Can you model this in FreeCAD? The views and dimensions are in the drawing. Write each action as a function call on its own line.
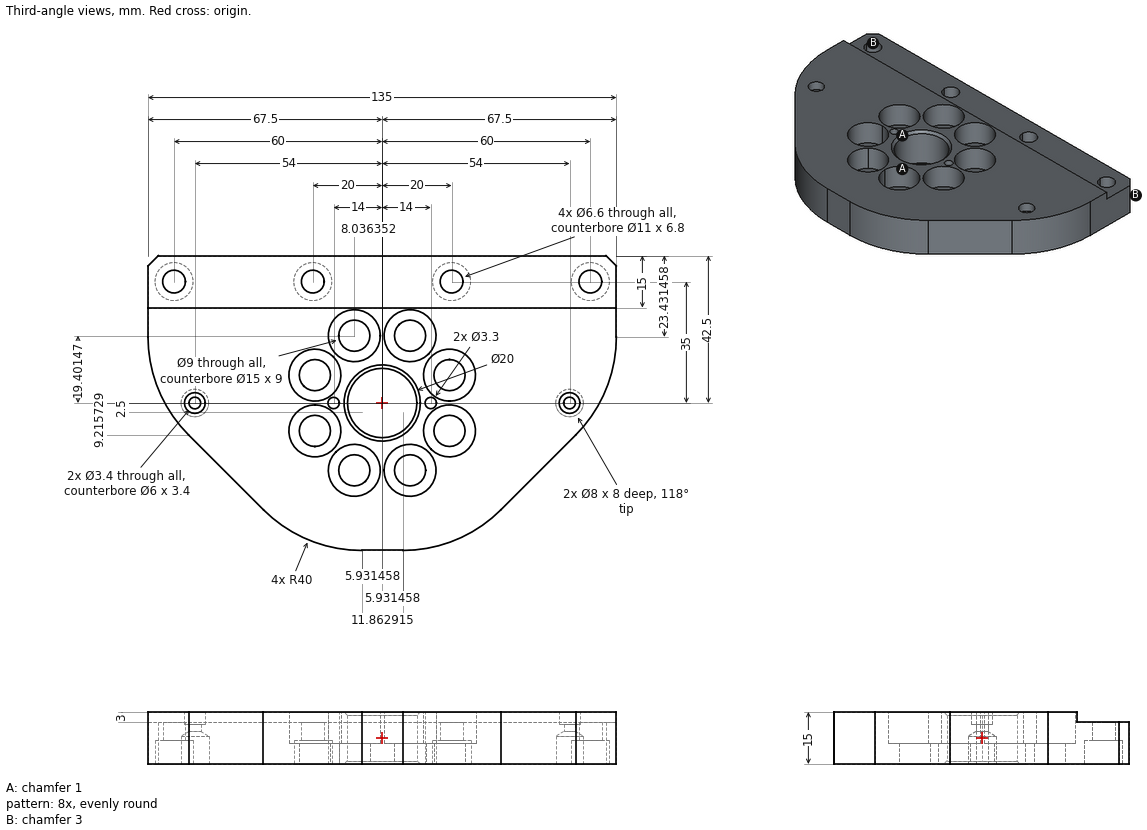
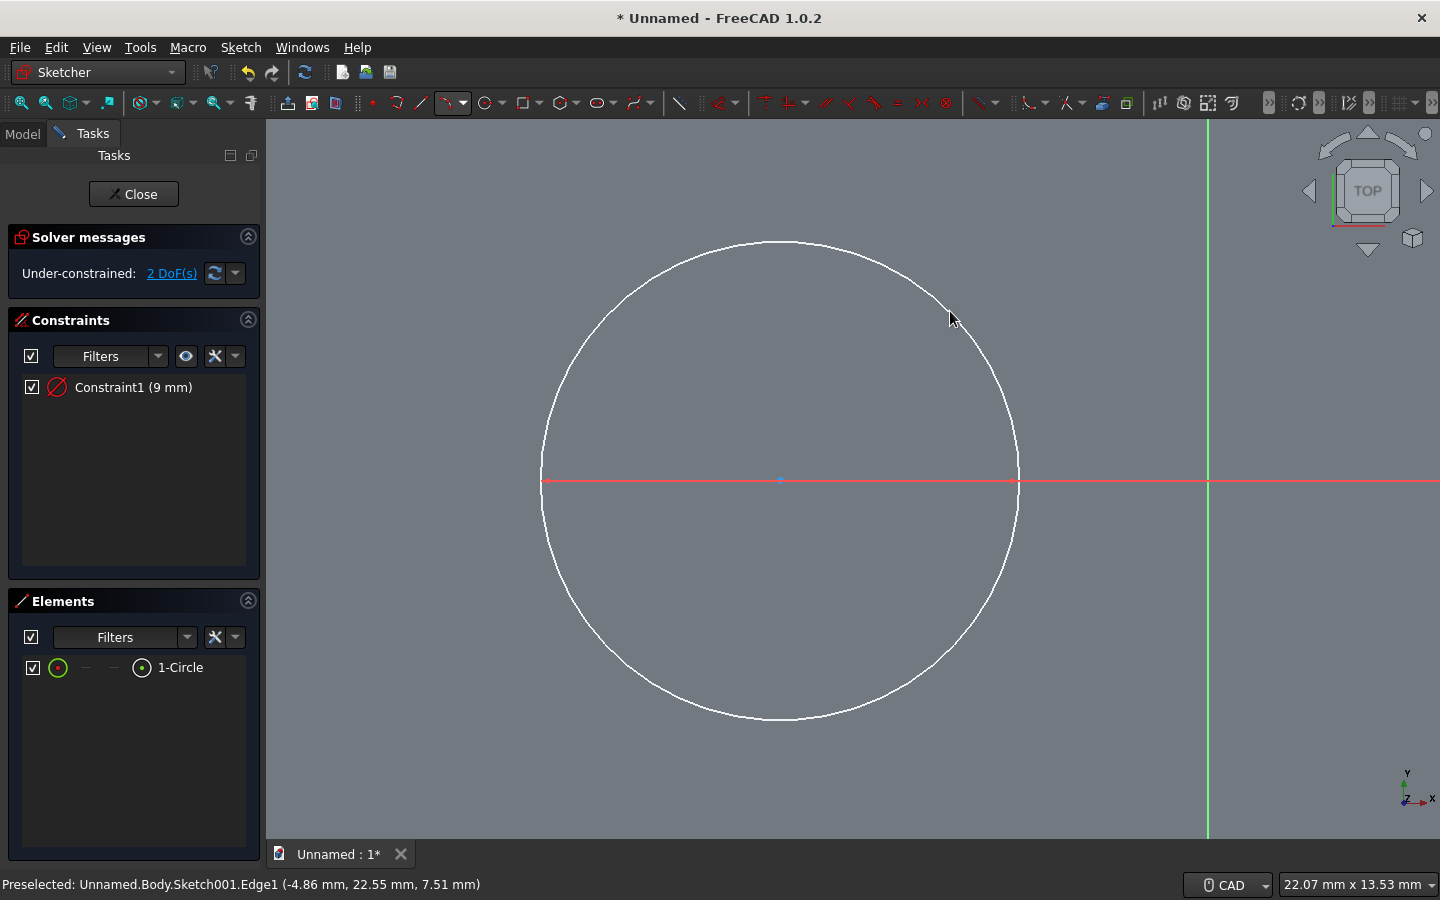
click(718, 104)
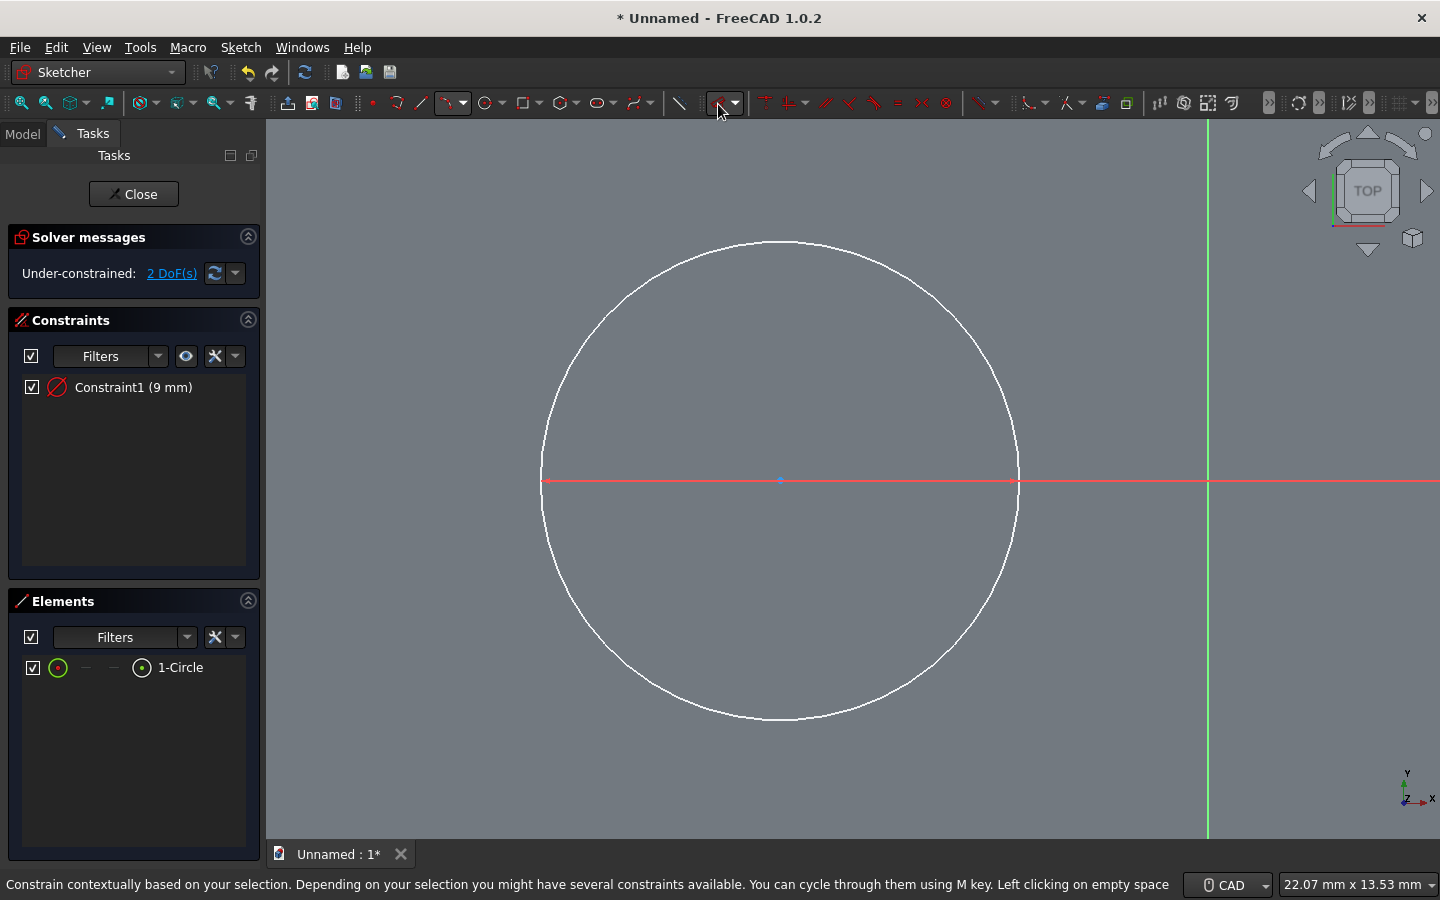
click(780, 481)
click(994, 447)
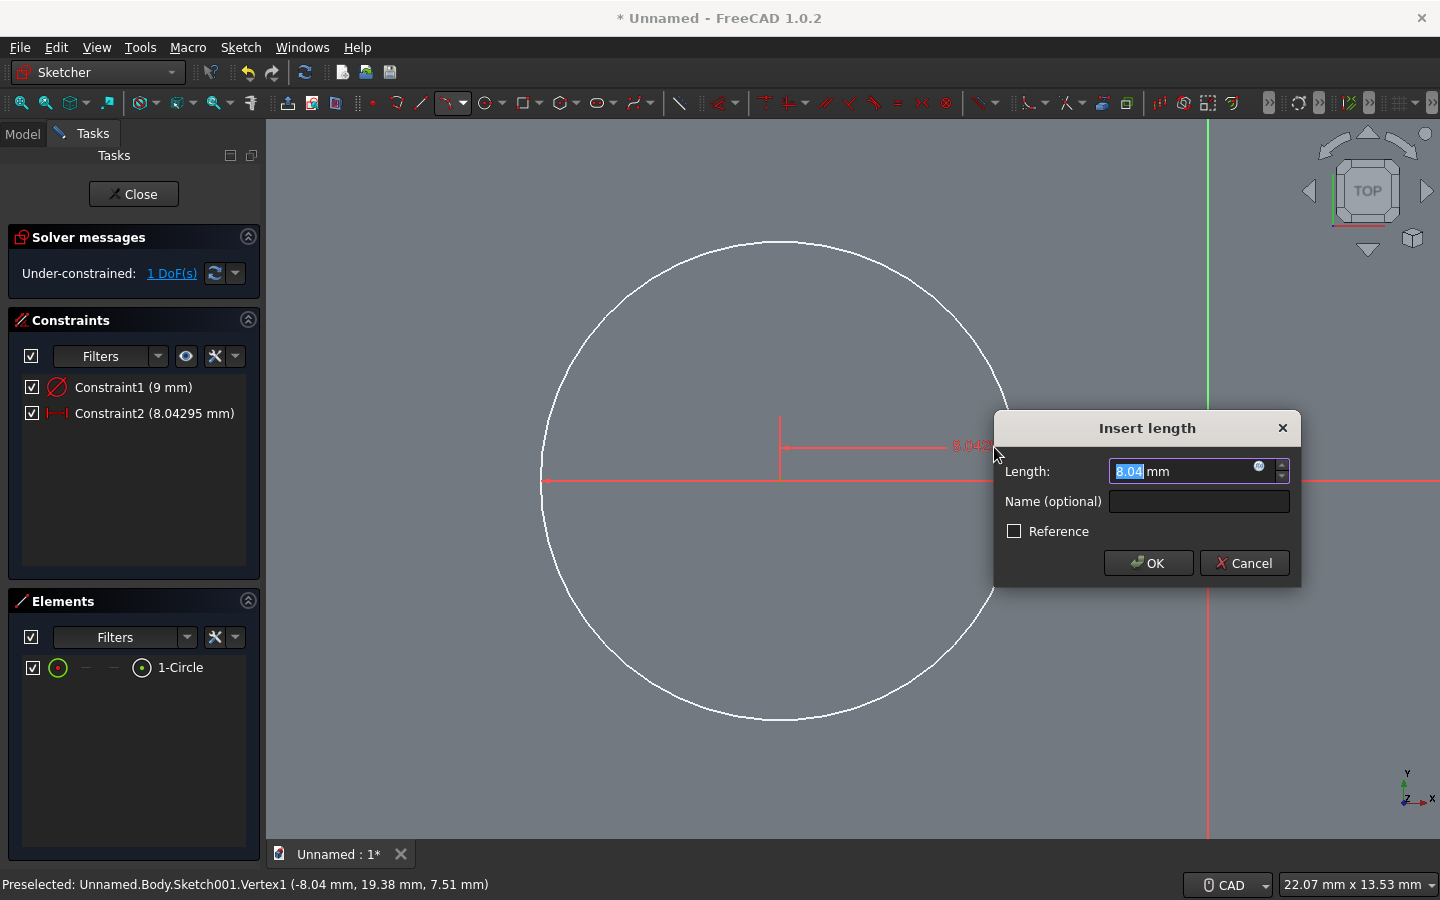
text(8.036352)
key(Return)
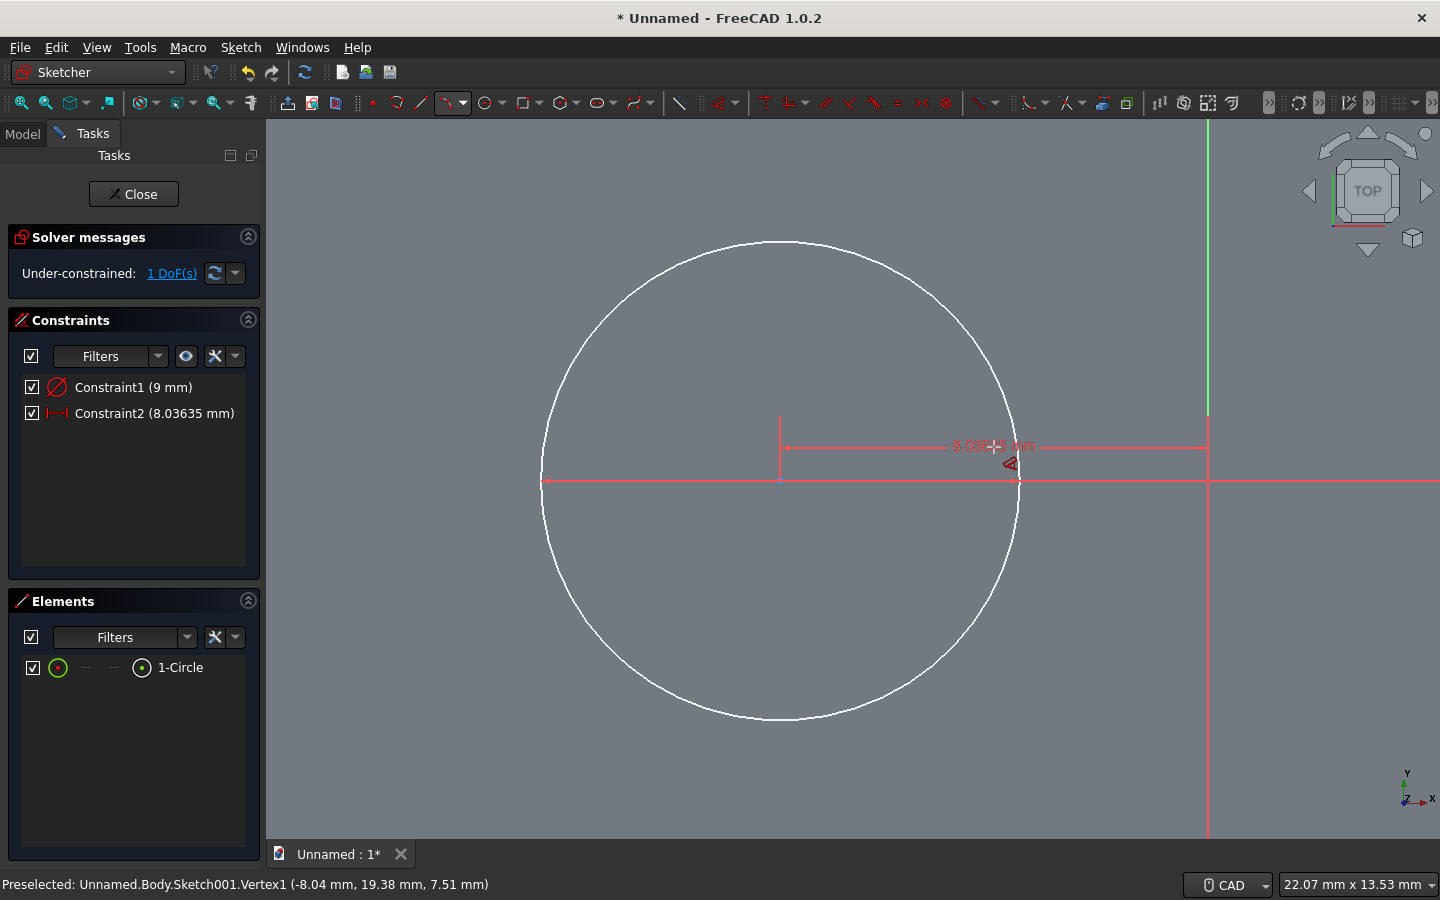
click(780, 481)
click(1242, 646)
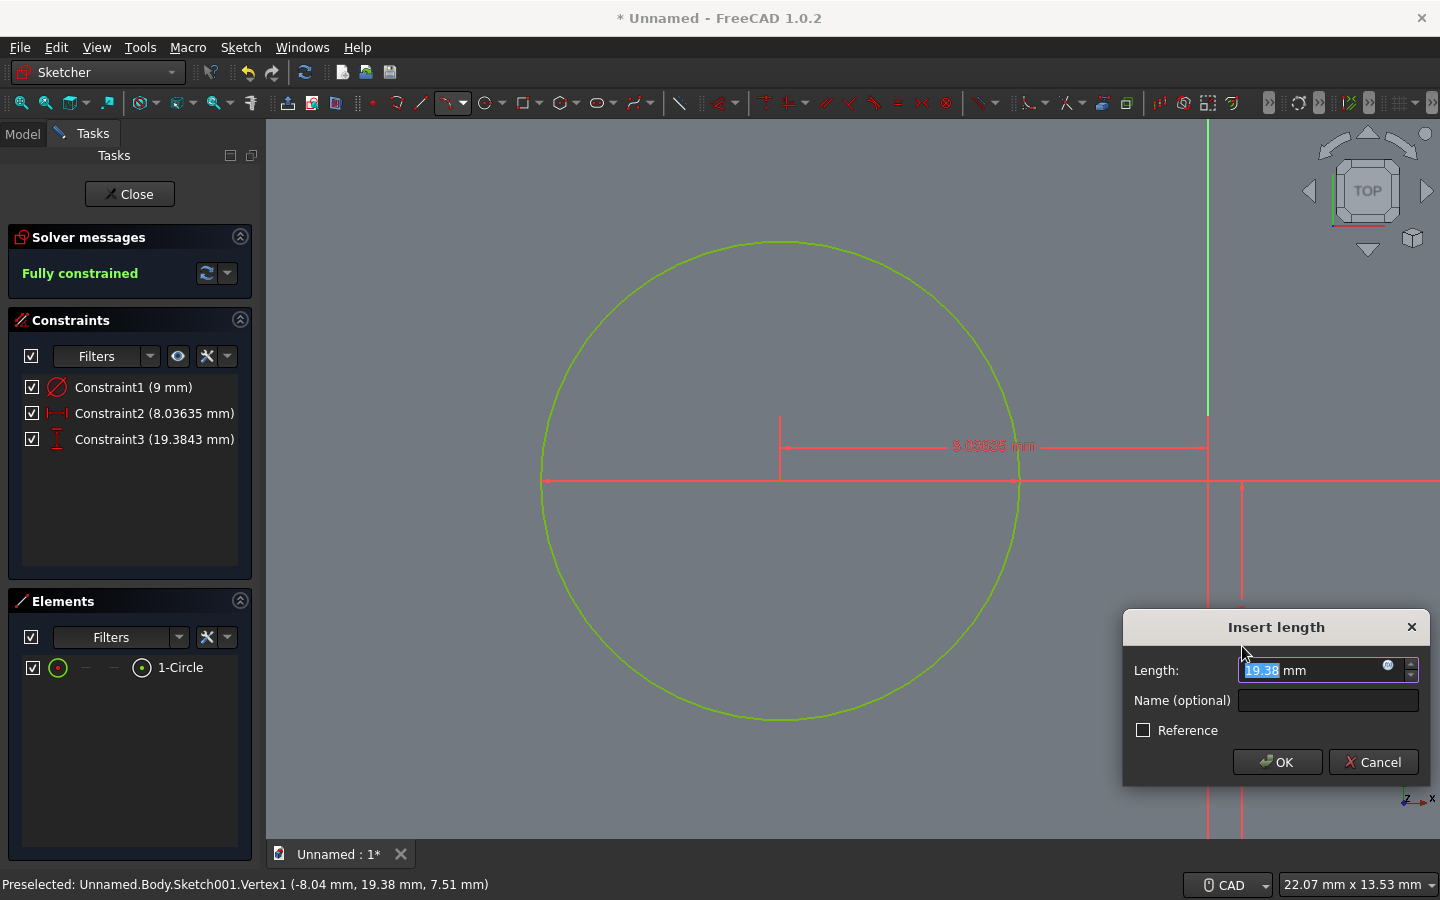
text(19.40147)
key(Return)
key(Escape)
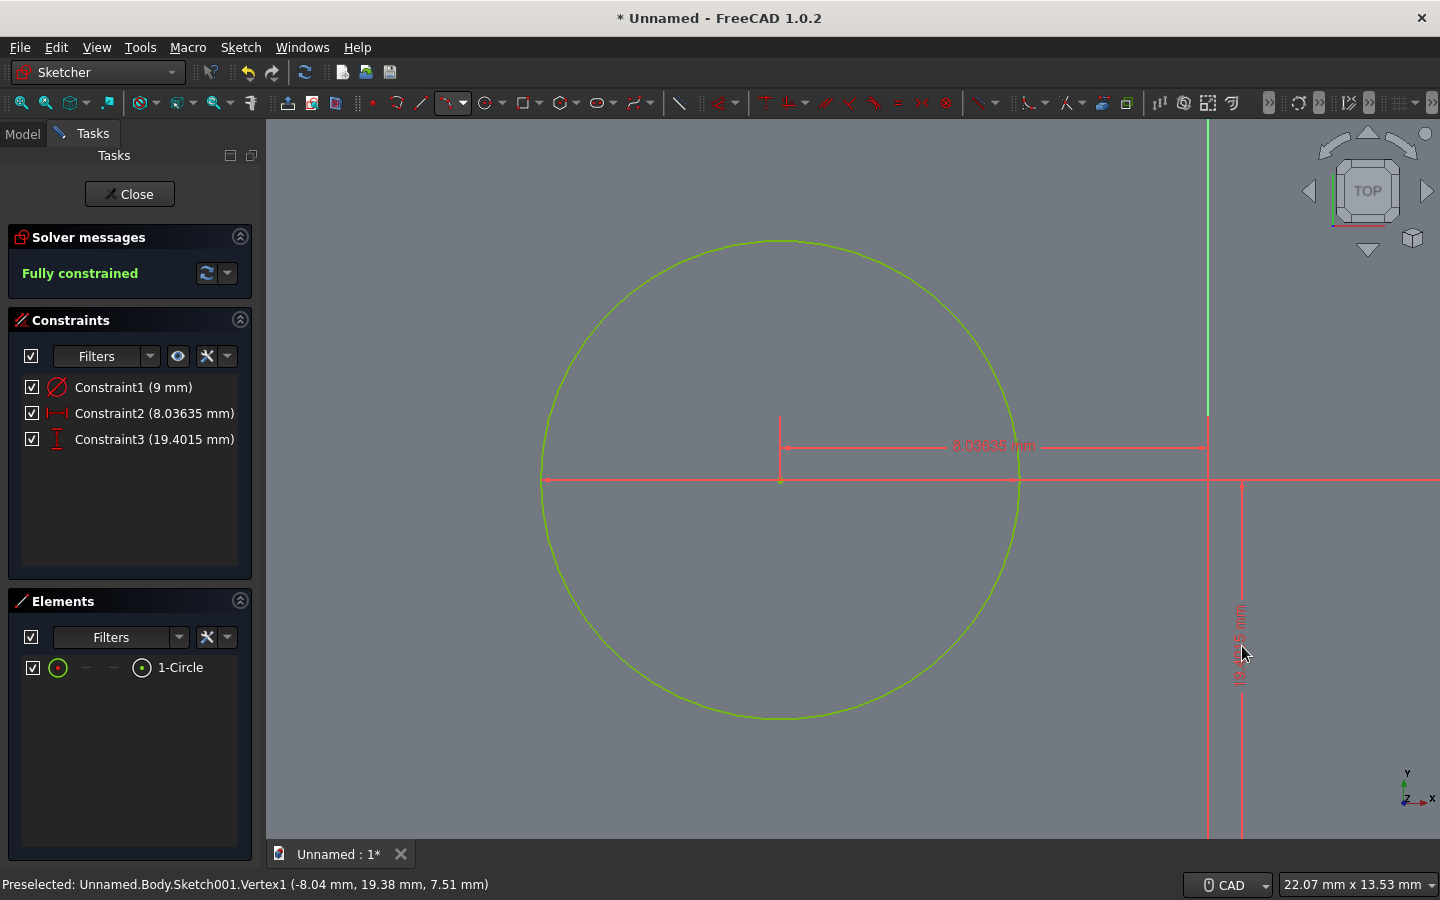
click(130, 194)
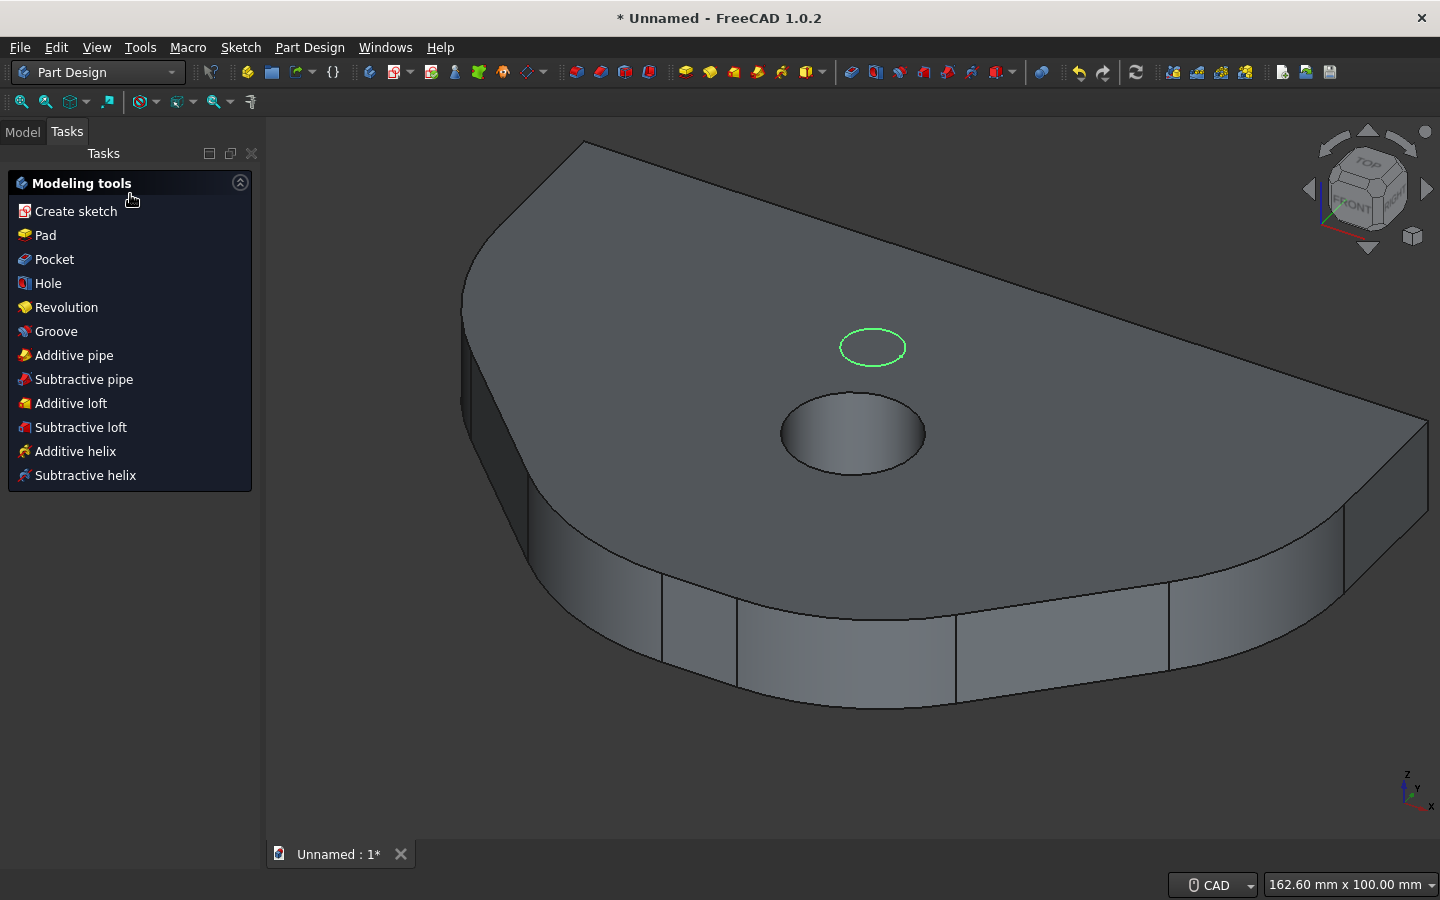
click(876, 72)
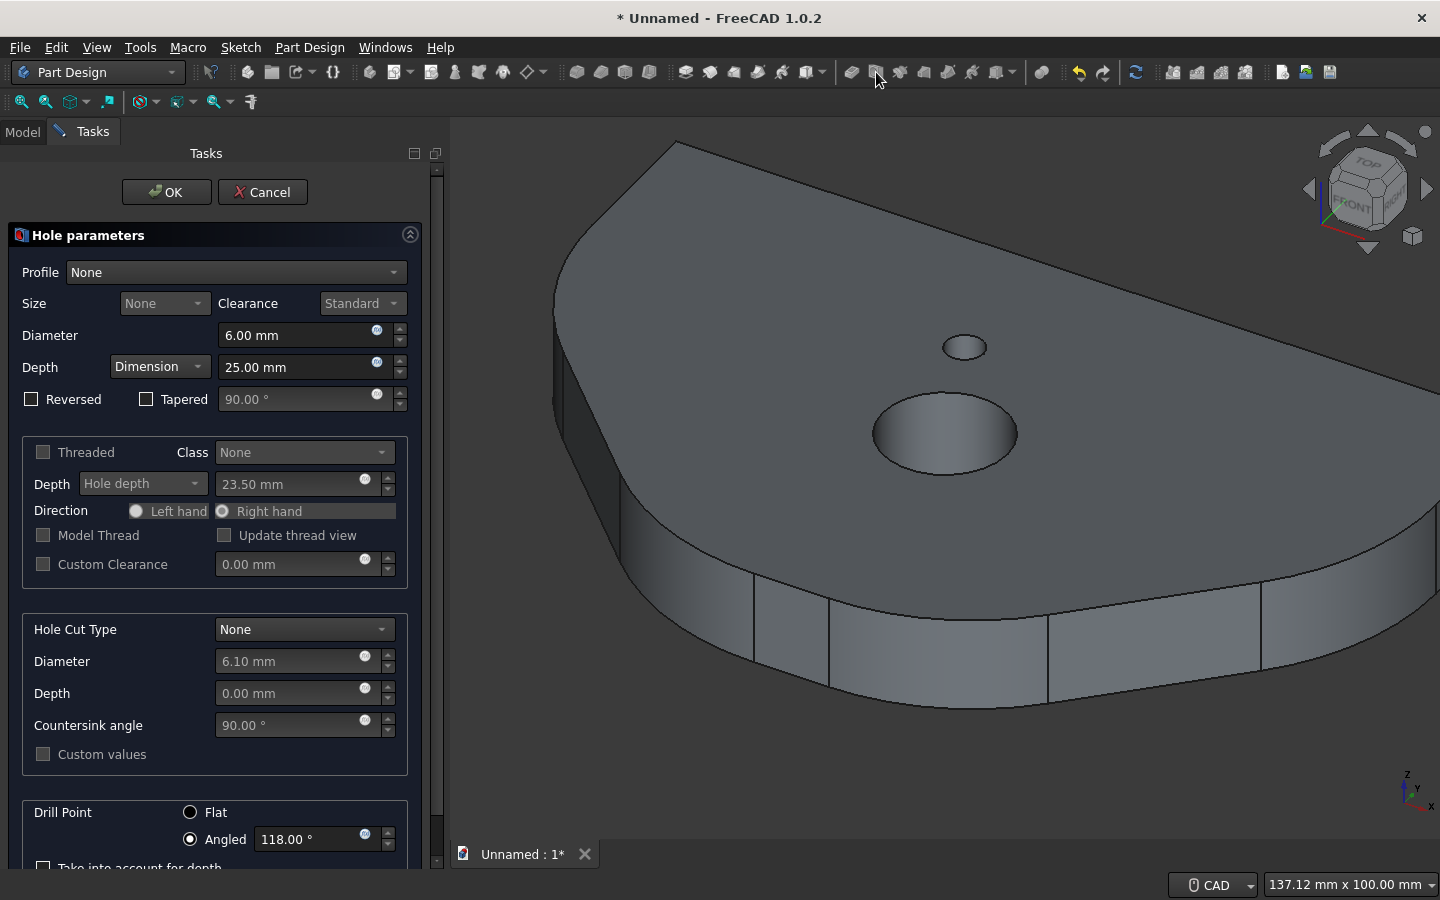
triple_click(305, 335)